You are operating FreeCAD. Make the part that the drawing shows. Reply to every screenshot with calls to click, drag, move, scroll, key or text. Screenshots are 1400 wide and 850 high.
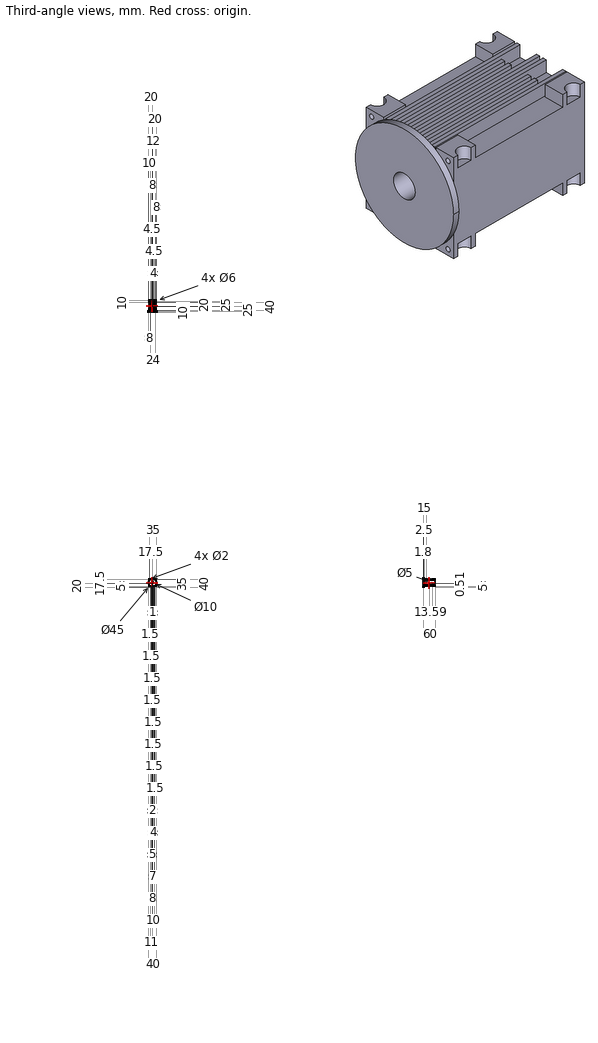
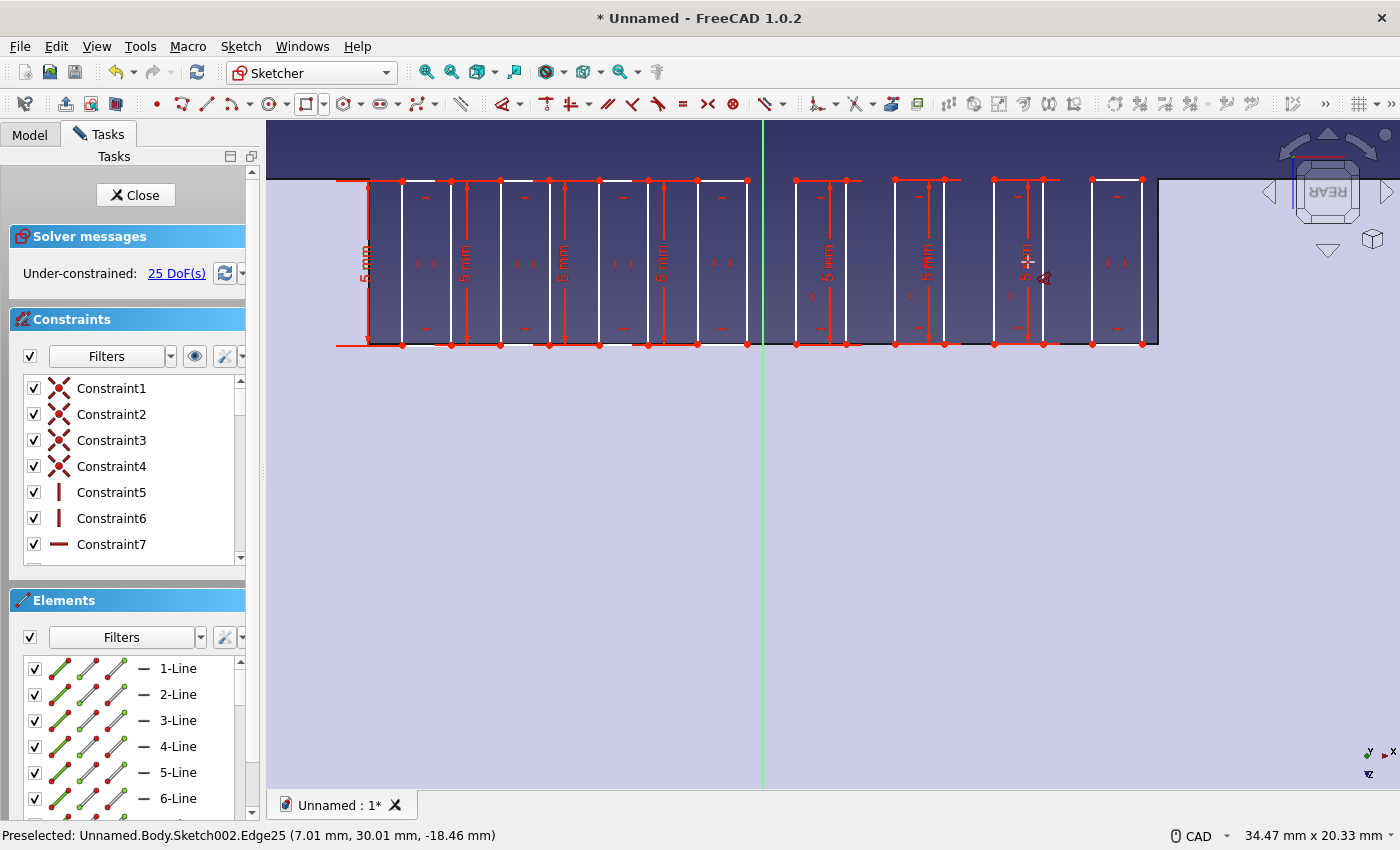
click(1092, 229)
click(1126, 262)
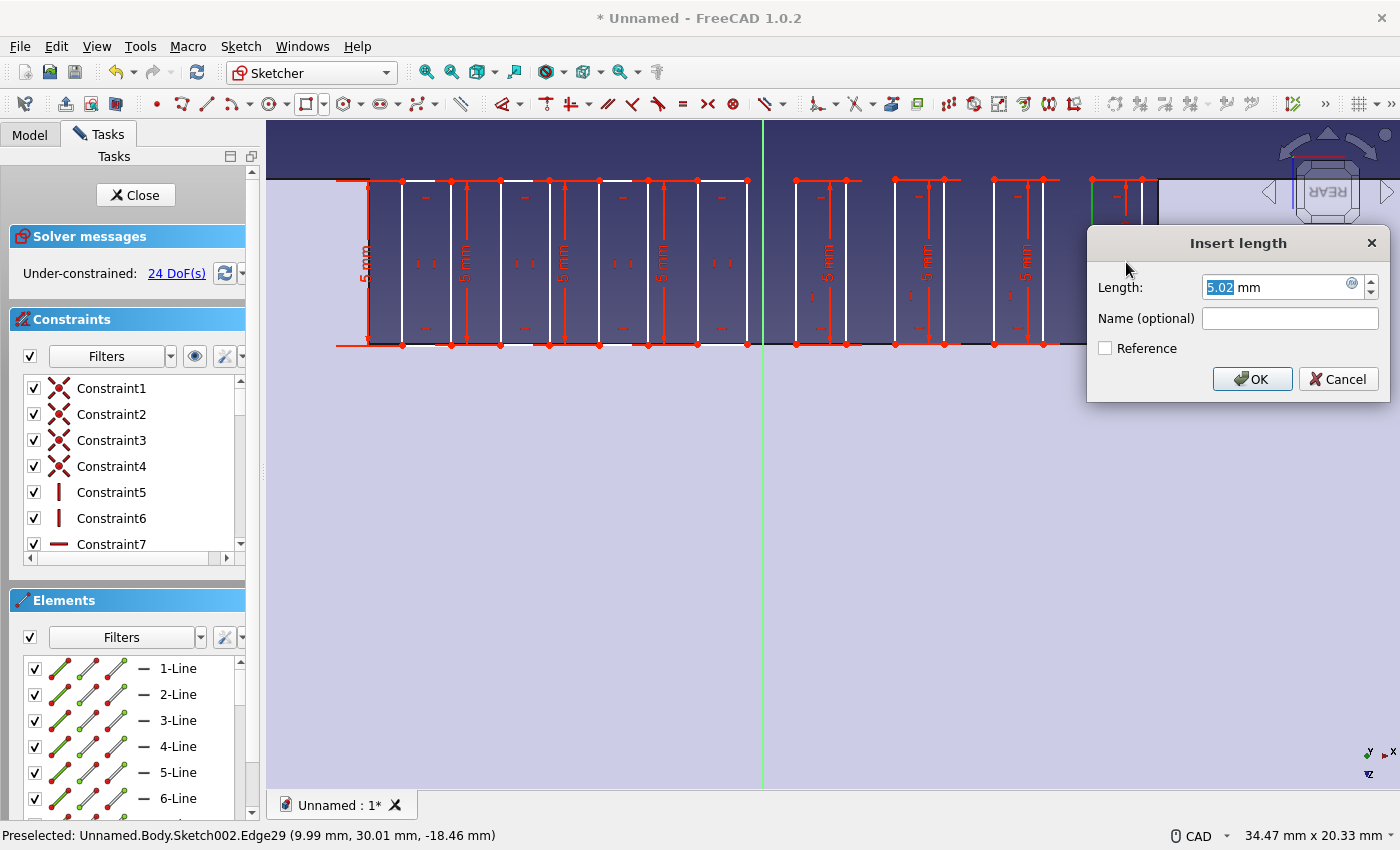
text(5)
key(Return)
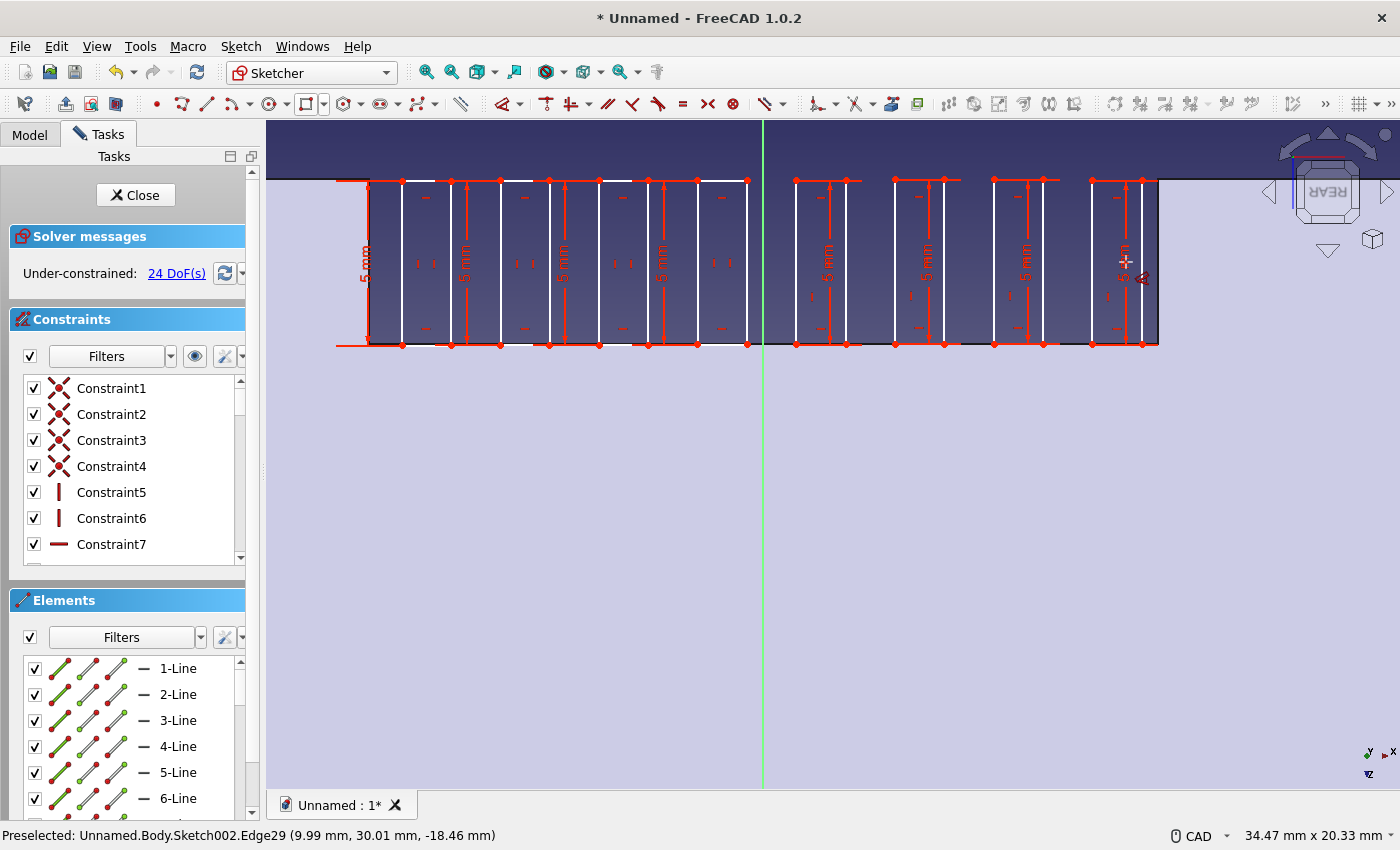
click(501, 181)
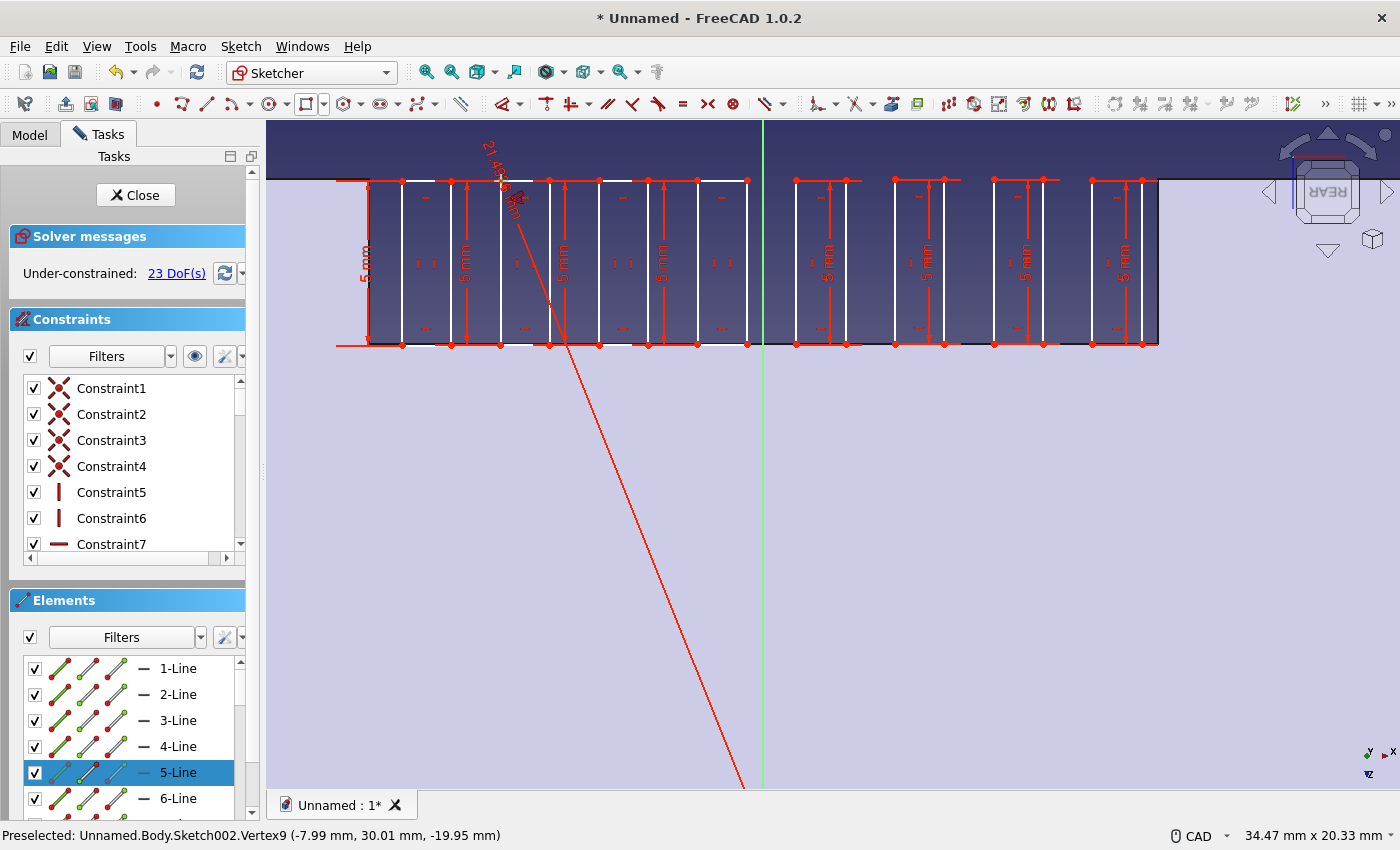
key(Escape)
key(Escape)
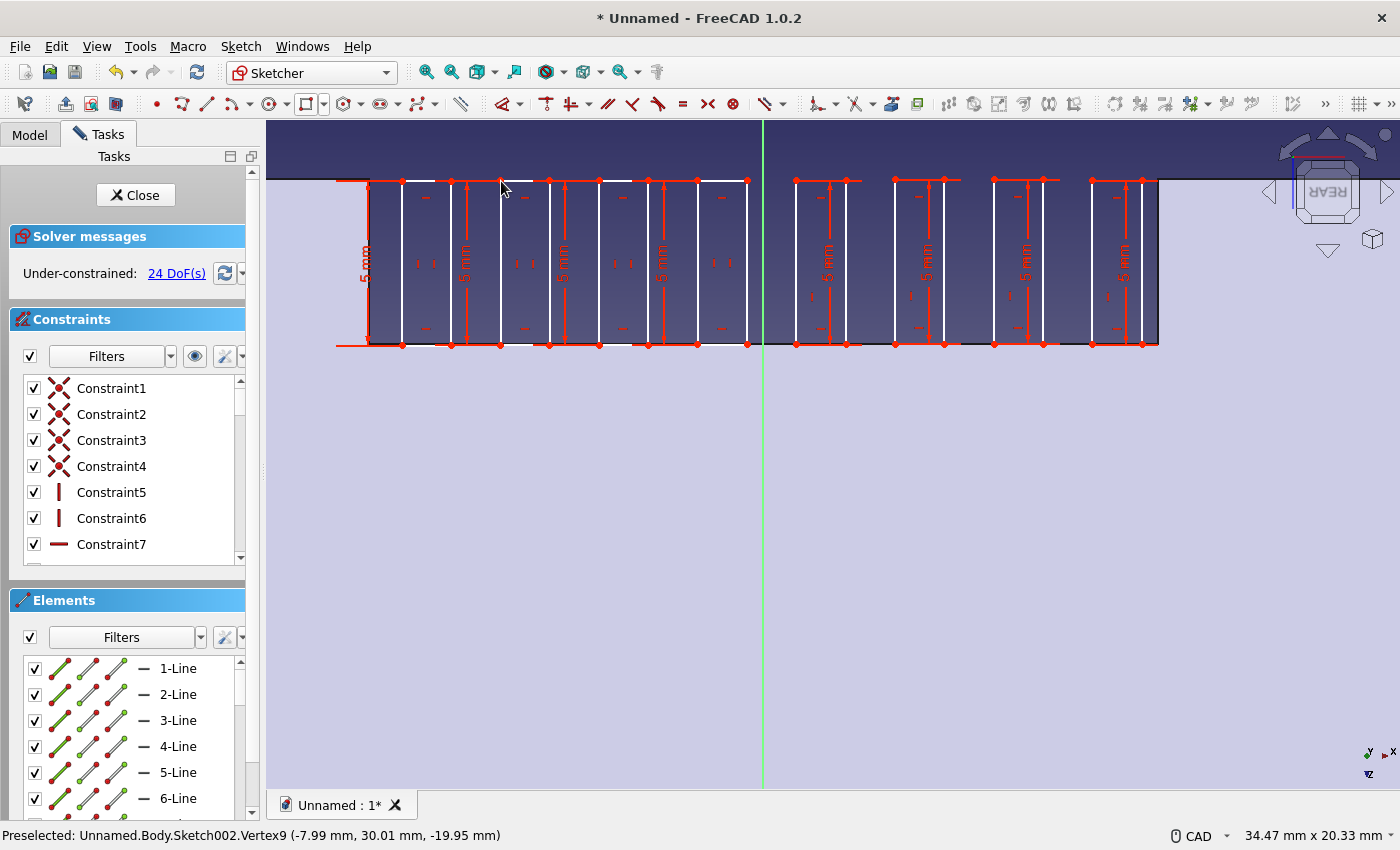
click(501, 181)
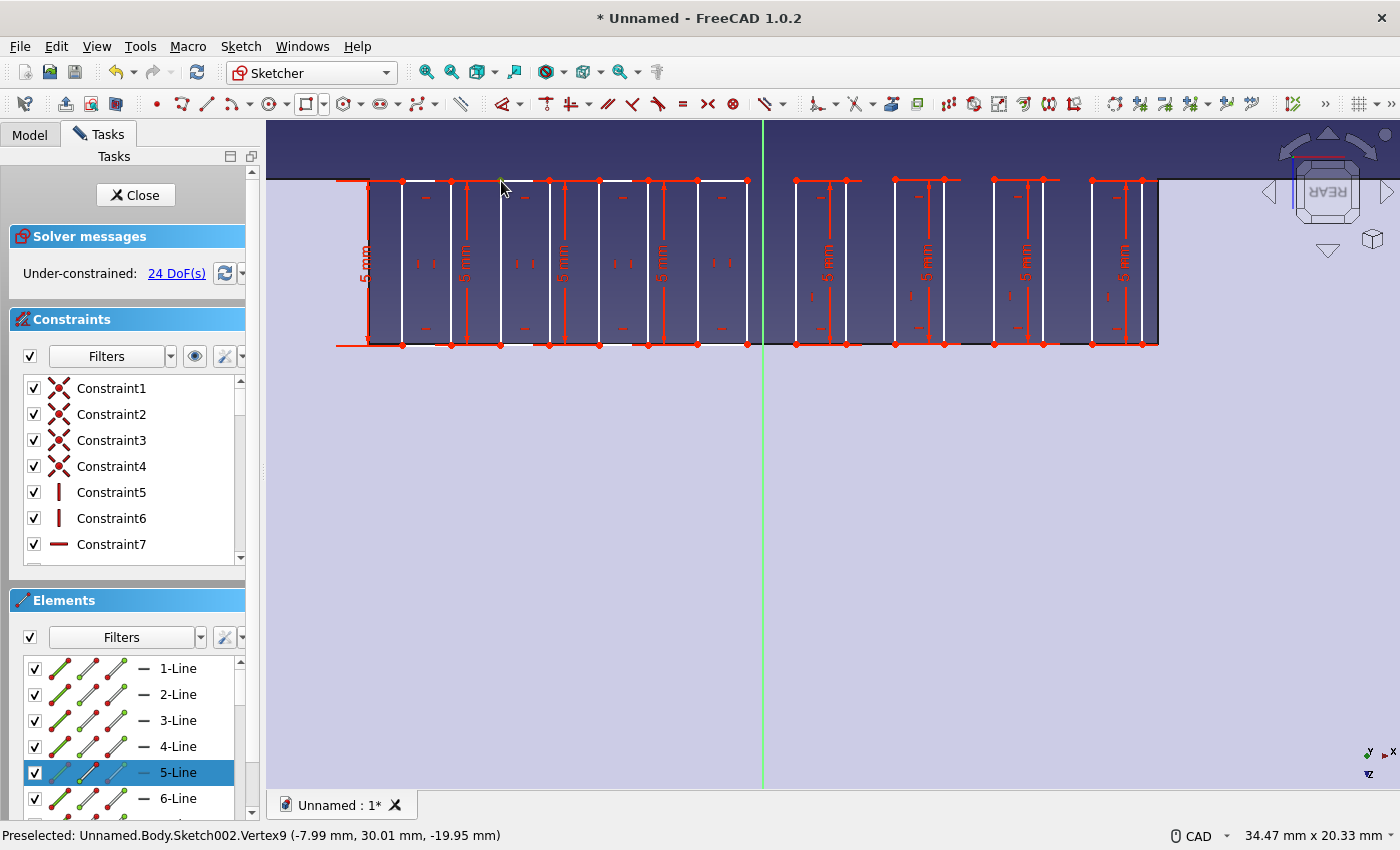
click(520, 104)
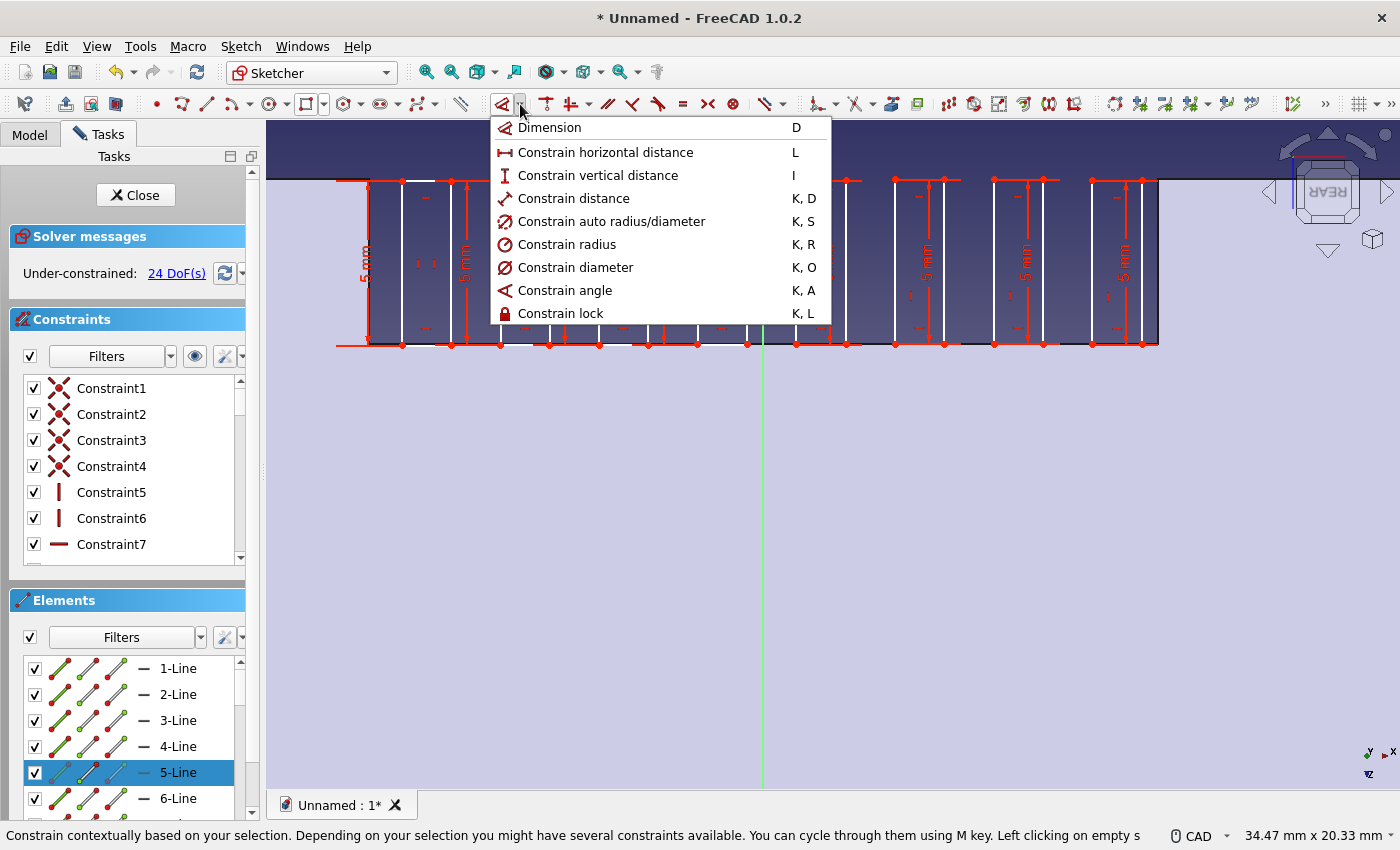
click(661, 152)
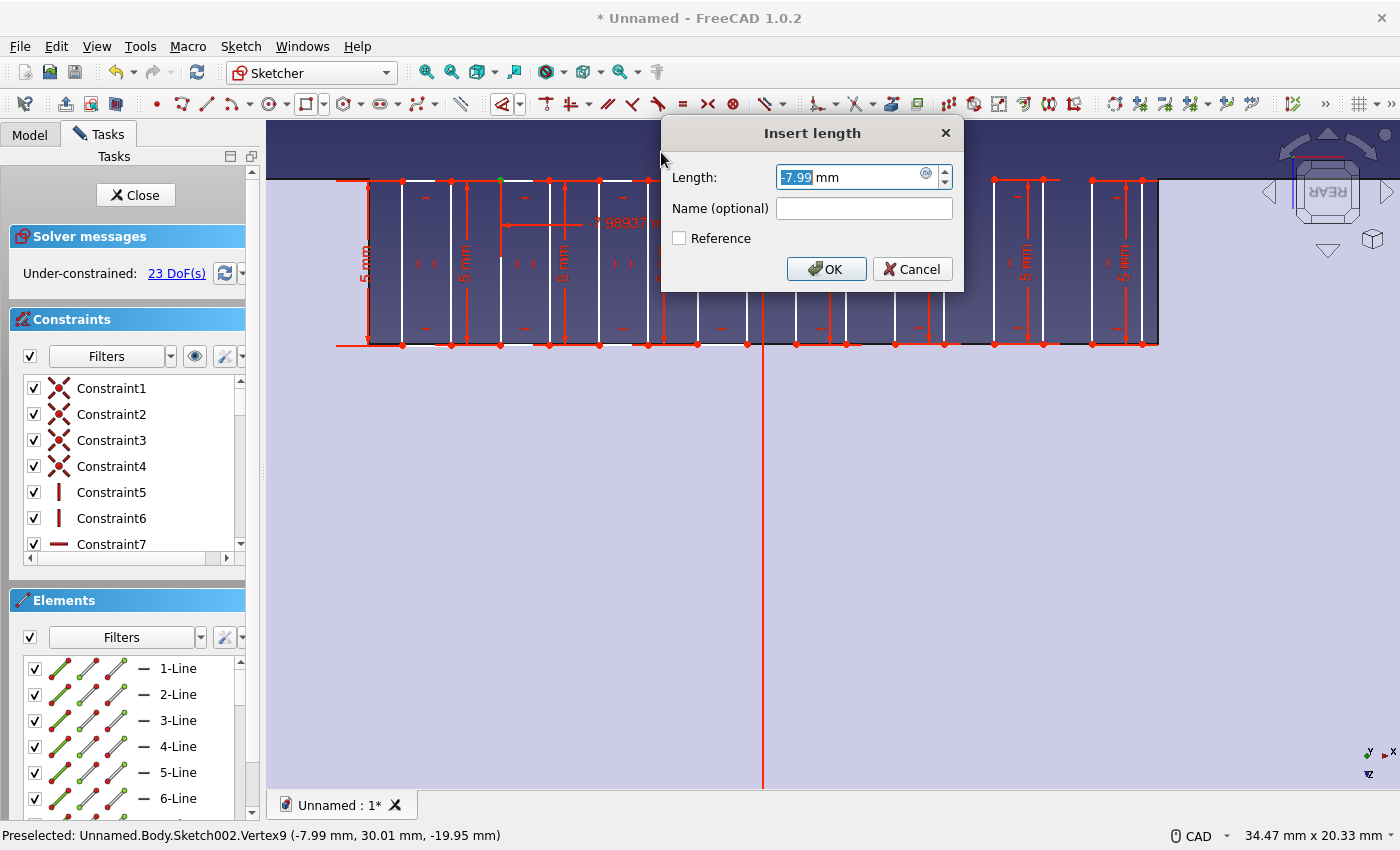
text(-8)
key(Return)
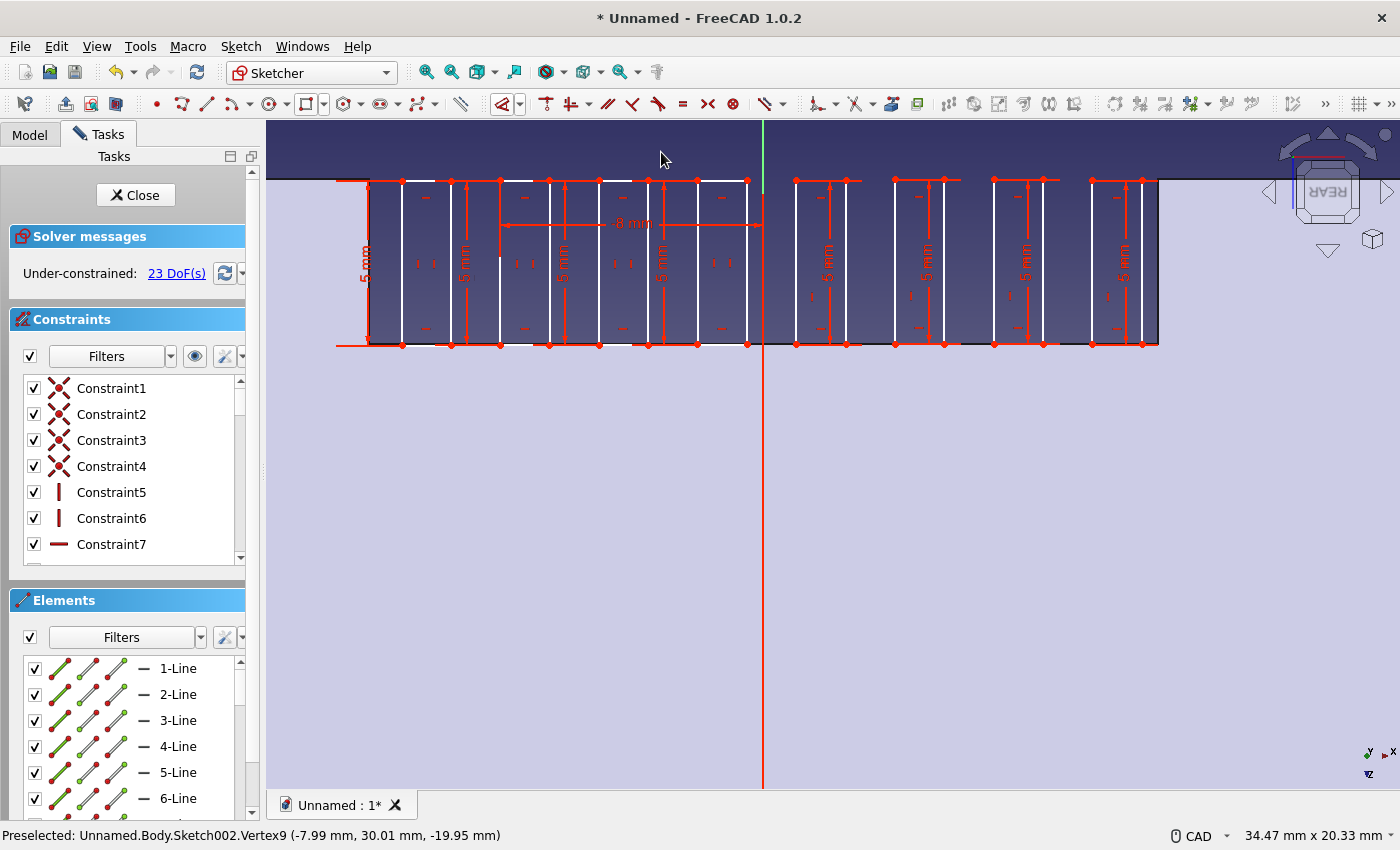
click(599, 181)